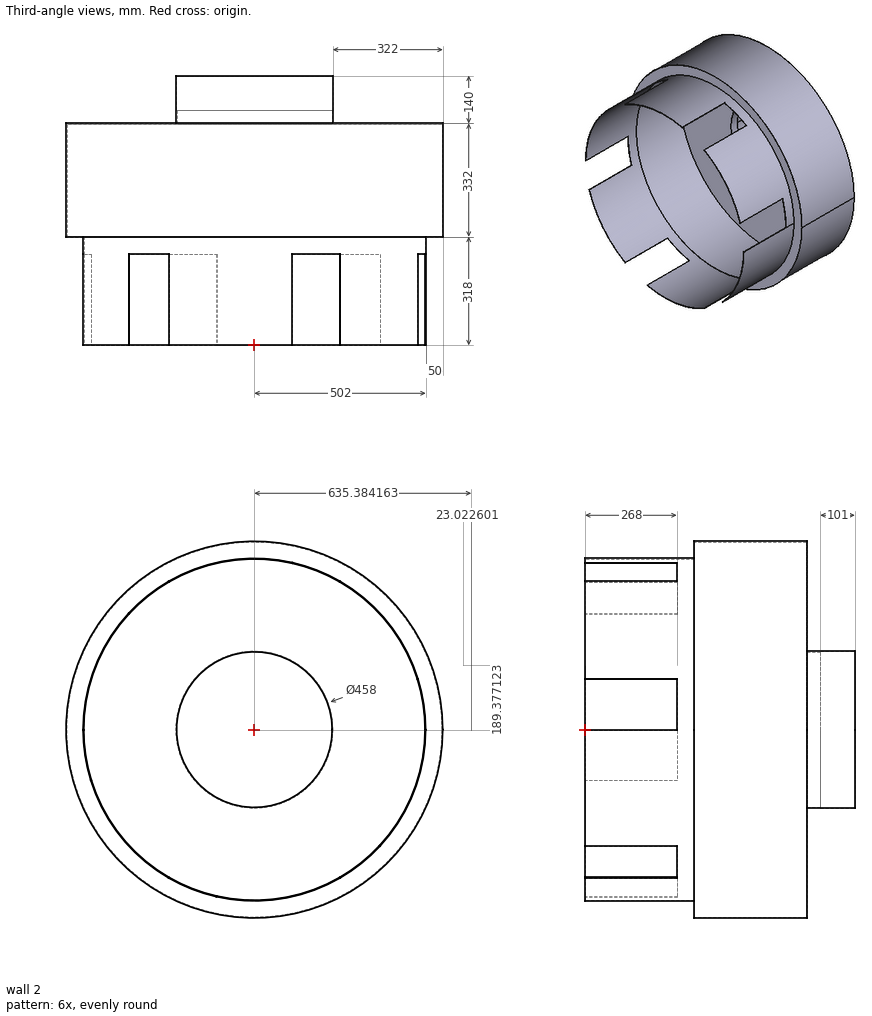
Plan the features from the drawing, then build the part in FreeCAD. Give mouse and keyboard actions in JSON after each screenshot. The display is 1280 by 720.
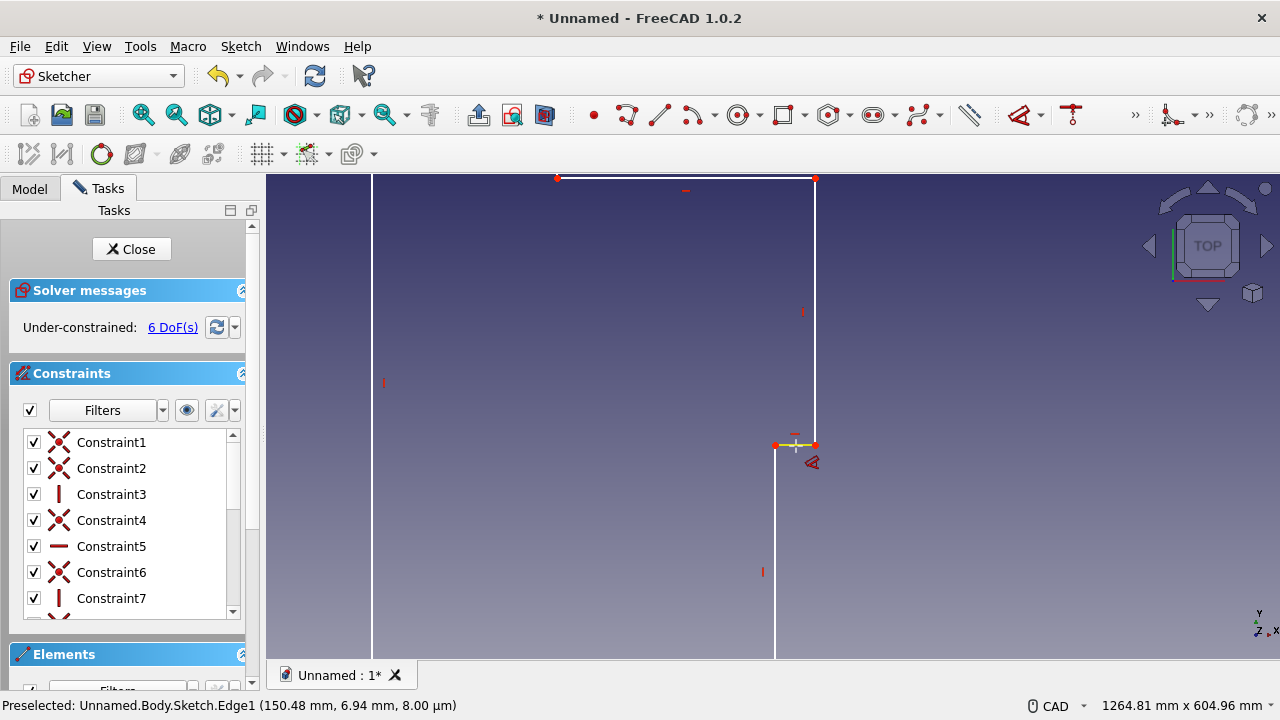
{"action": "left_click", "coordinate": [795, 445]}
{"action": "left_click", "coordinate": [795, 479]}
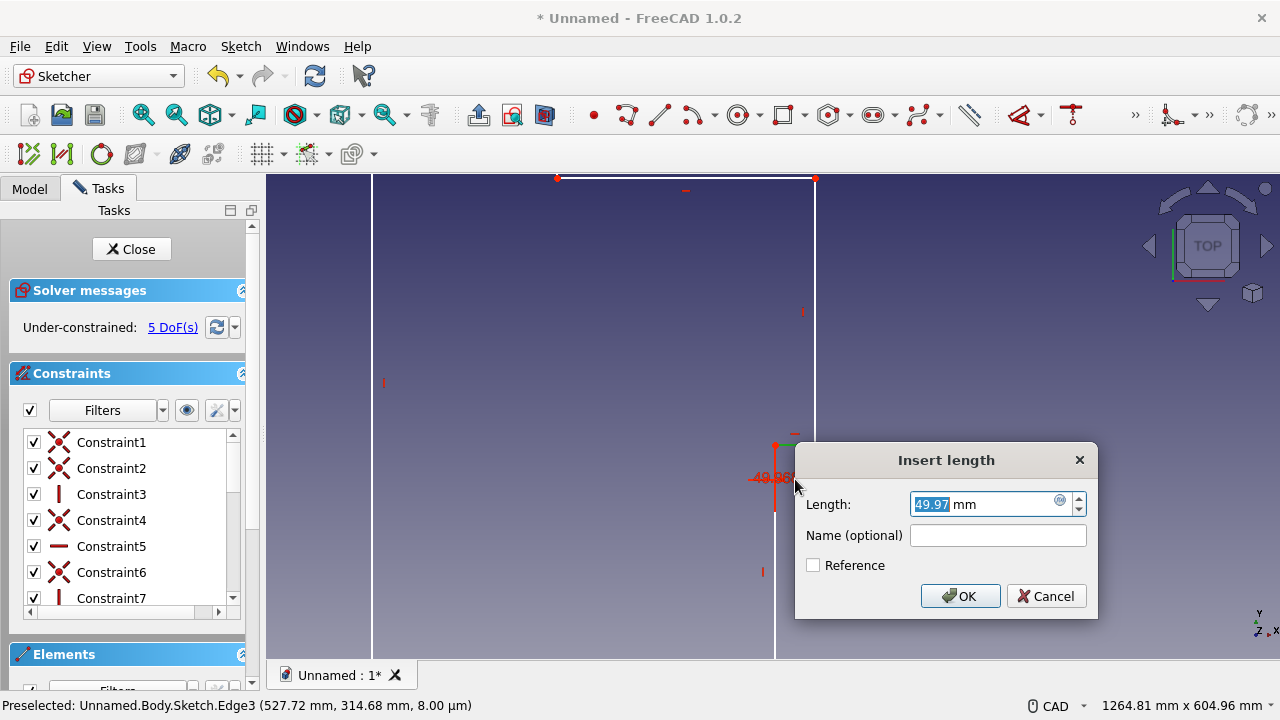
{"action": "type", "text": "50"}
{"action": "key", "text": "Return"}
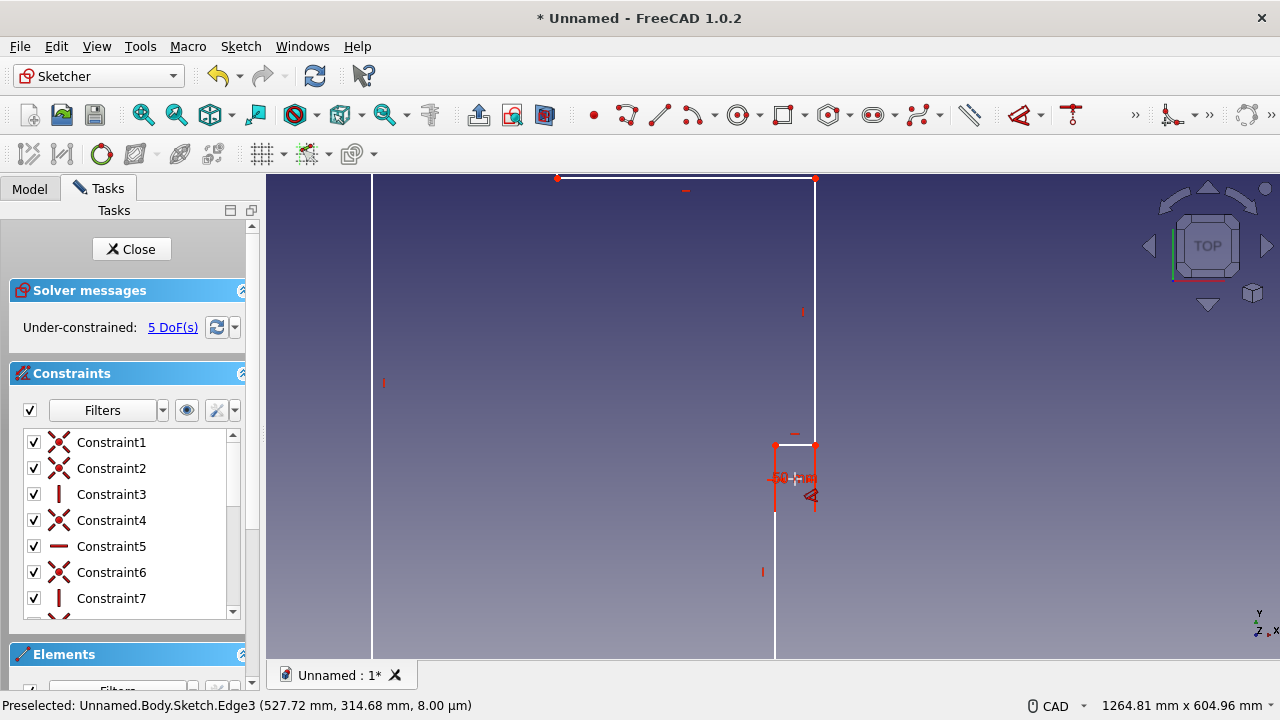
{"action": "scroll", "coordinate": [795, 446], "scroll_direction": "down", "scroll_amount": 4}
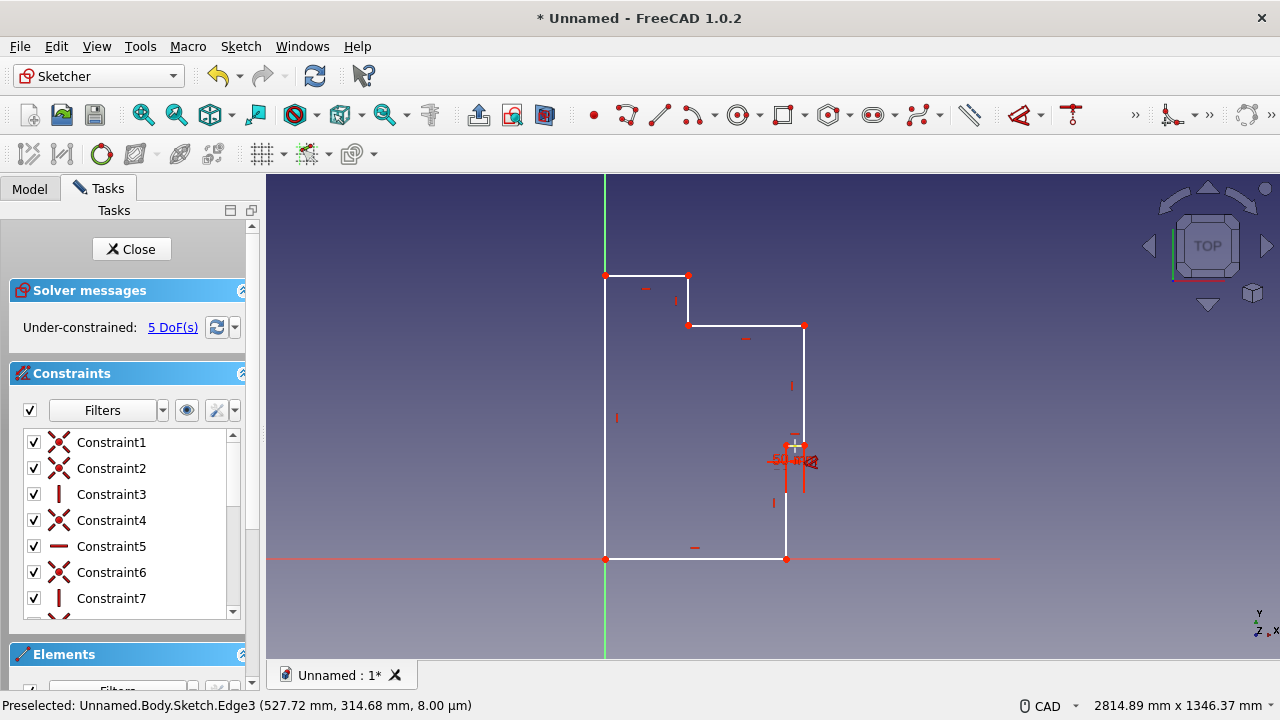
{"action": "left_click", "coordinate": [660, 559]}
{"action": "left_click", "coordinate": [696, 593]}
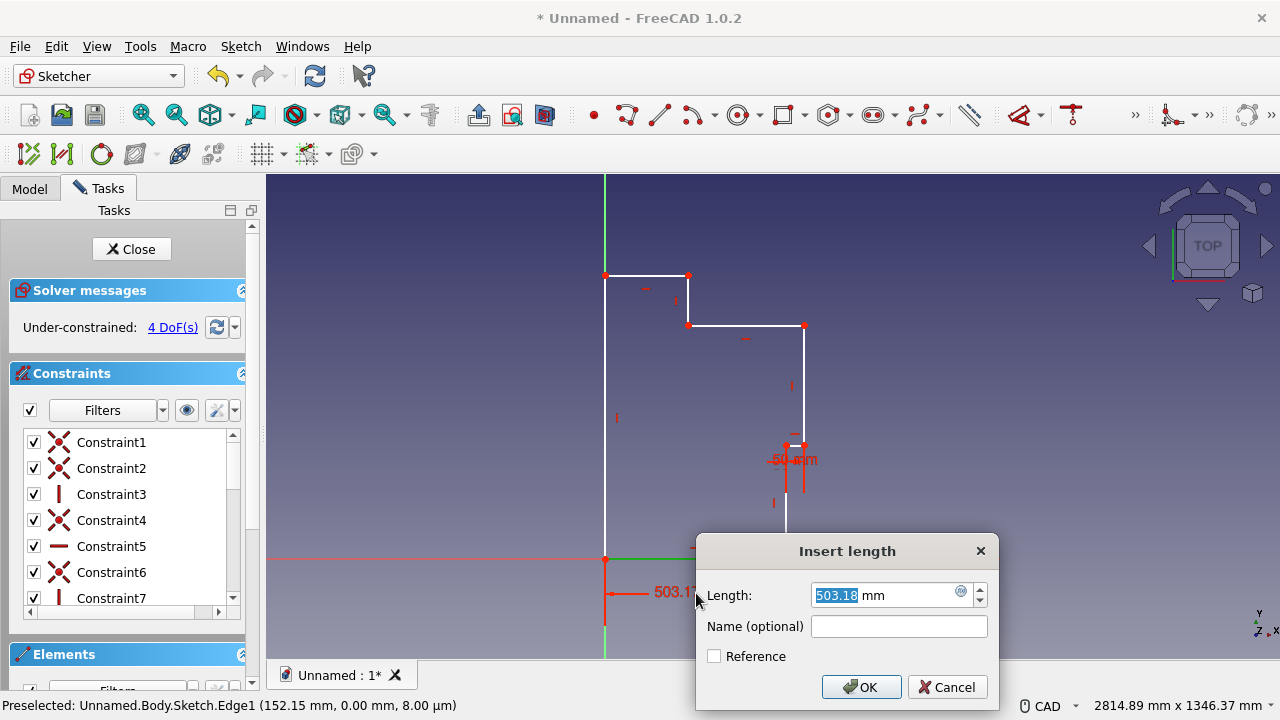
{"action": "type", "text": "502"}
{"action": "key", "text": "Return"}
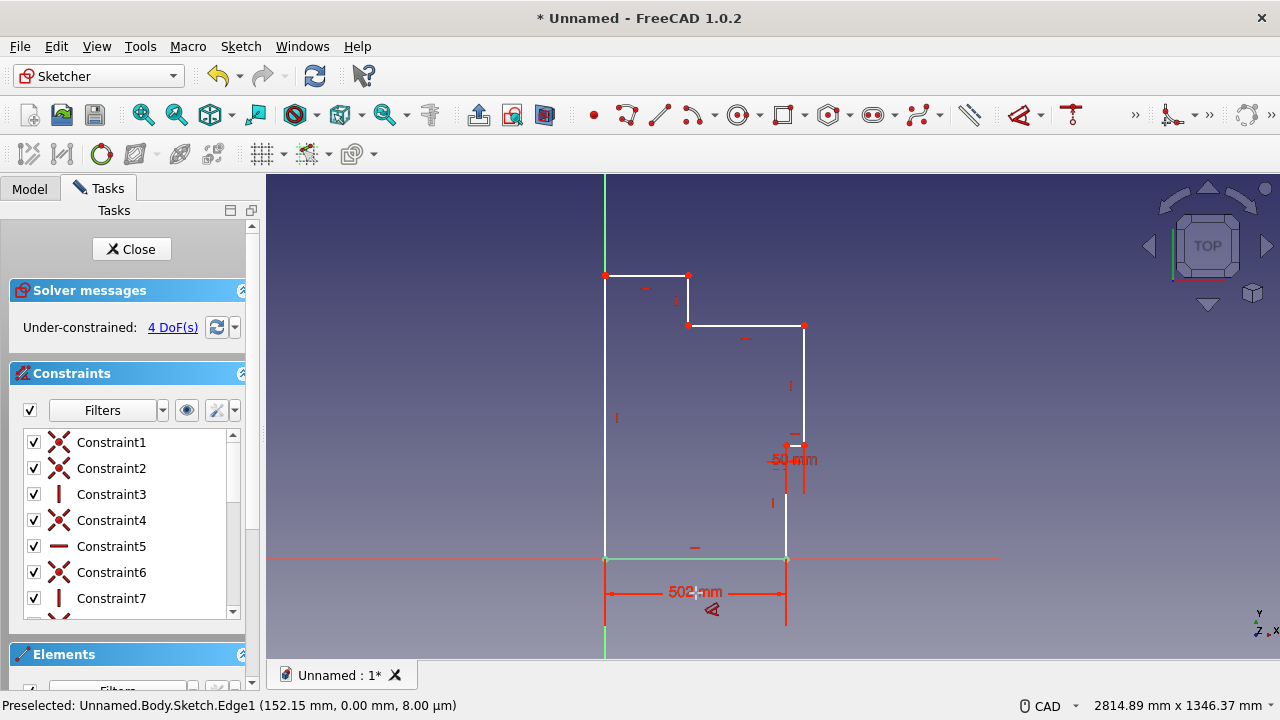
{"action": "left_click", "coordinate": [786, 525]}
{"action": "left_click", "coordinate": [820, 503]}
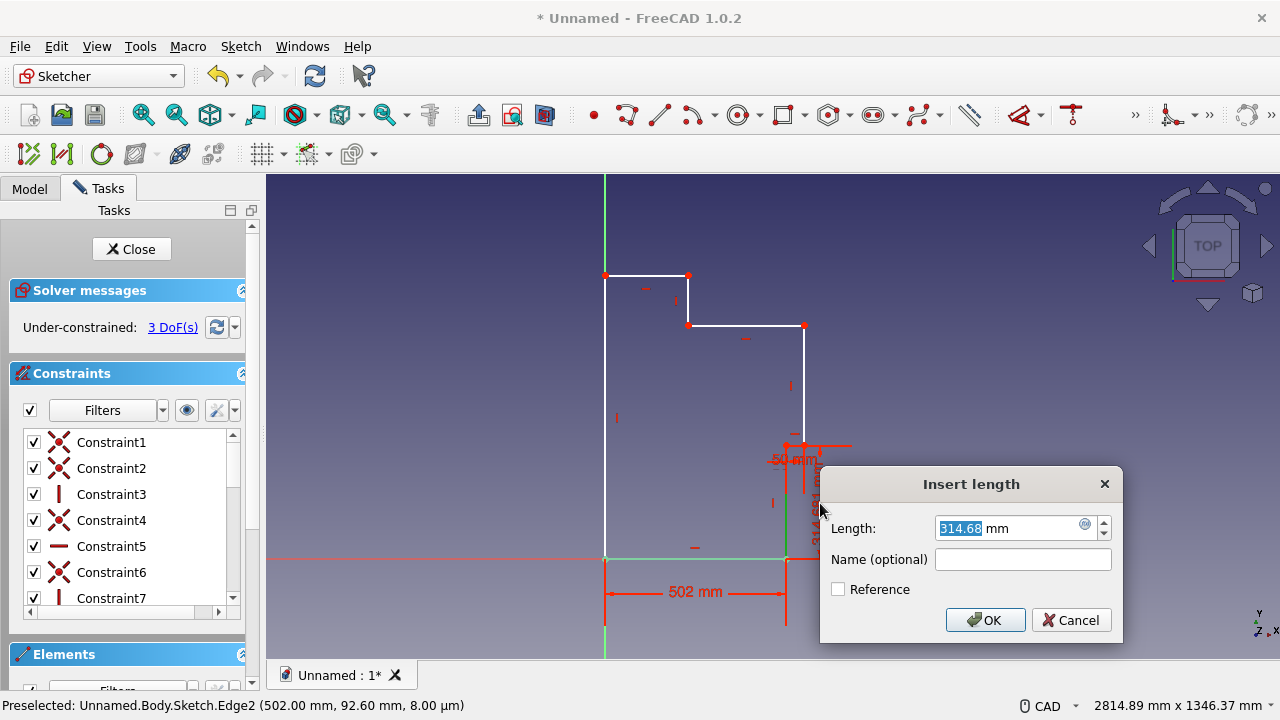
{"action": "type", "text": "318"}
{"action": "key", "text": "Return"}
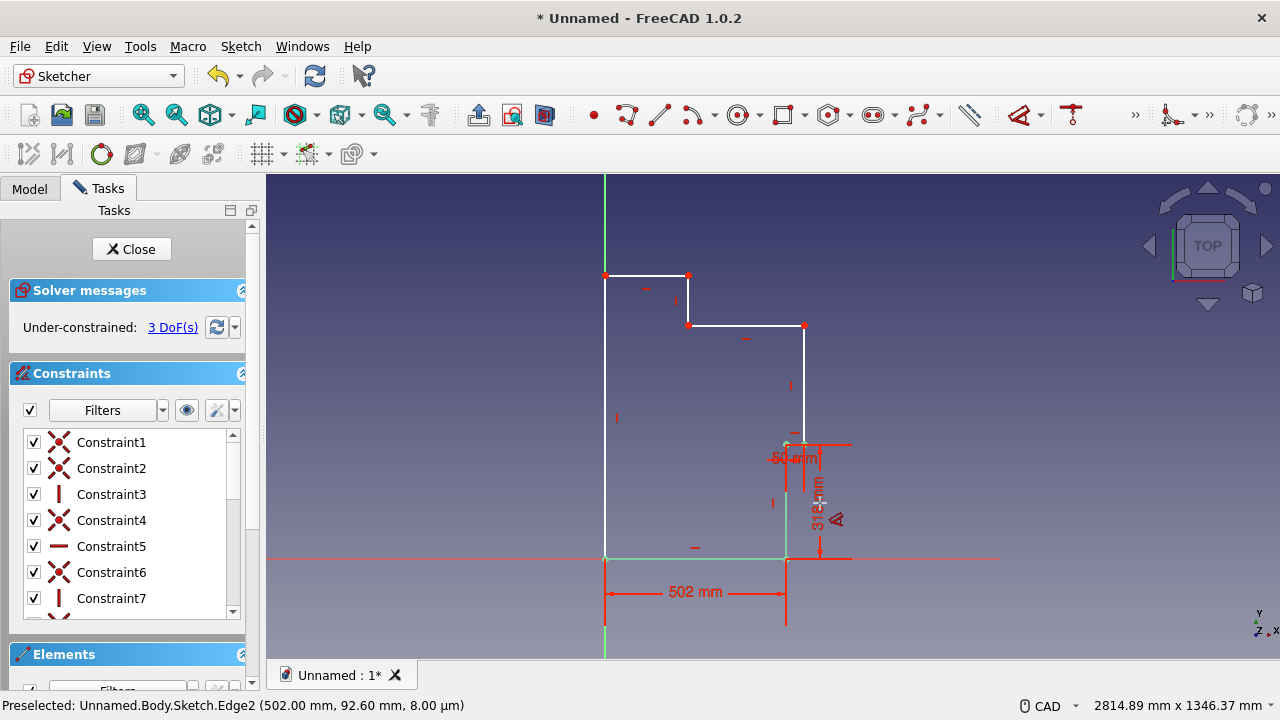
{"action": "left_click", "coordinate": [804, 409]}
{"action": "left_click", "coordinate": [838, 385]}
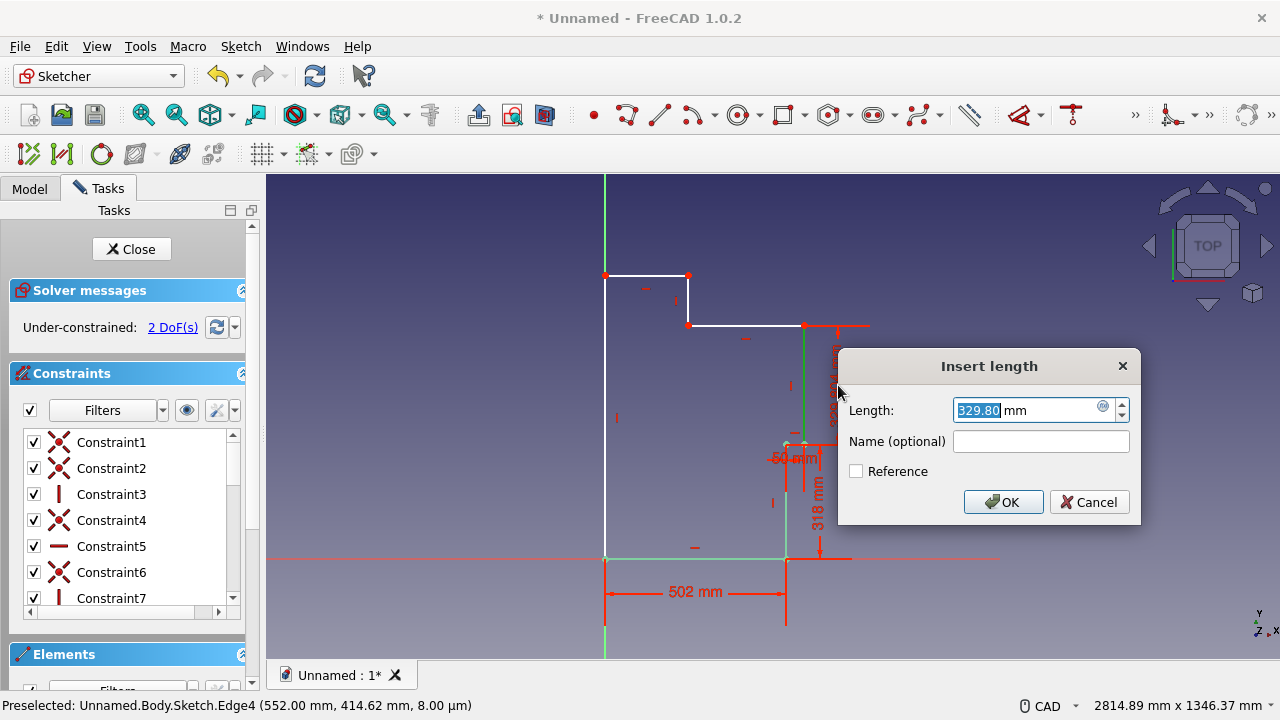
{"action": "type", "text": "332"}
{"action": "key", "text": "Return"}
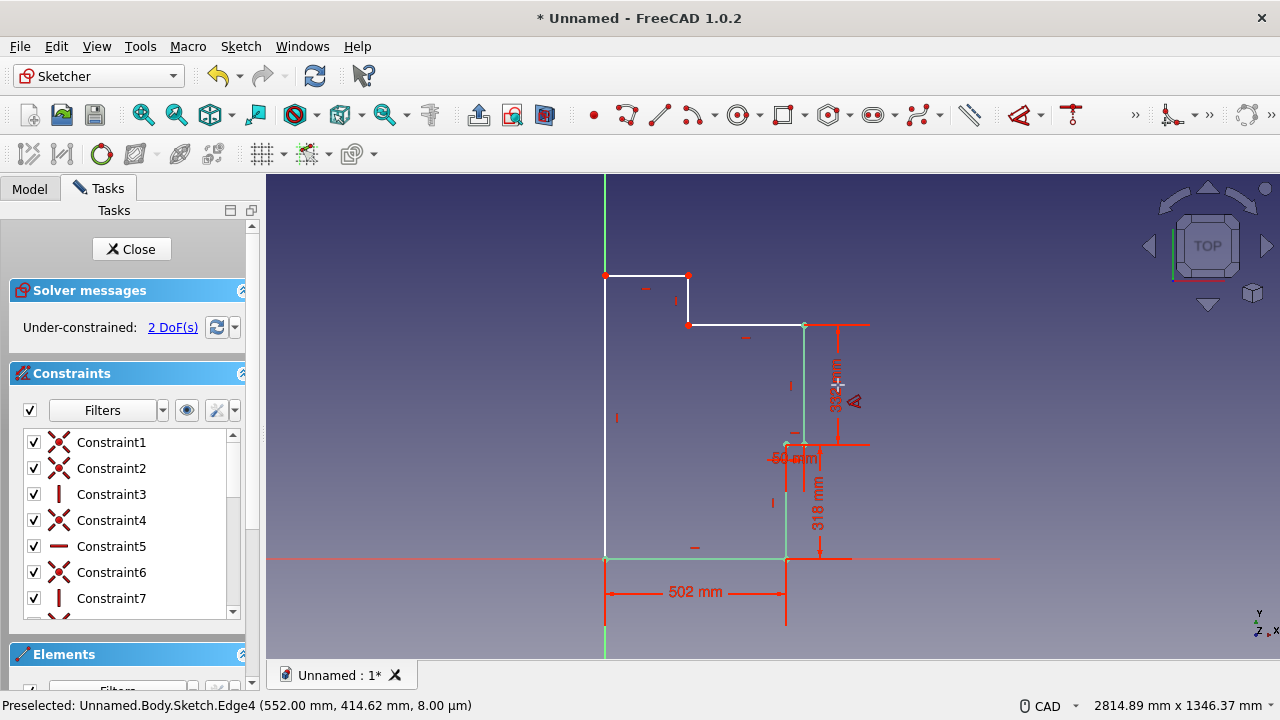
{"action": "left_click", "coordinate": [769, 325]}
{"action": "left_click", "coordinate": [746, 291]}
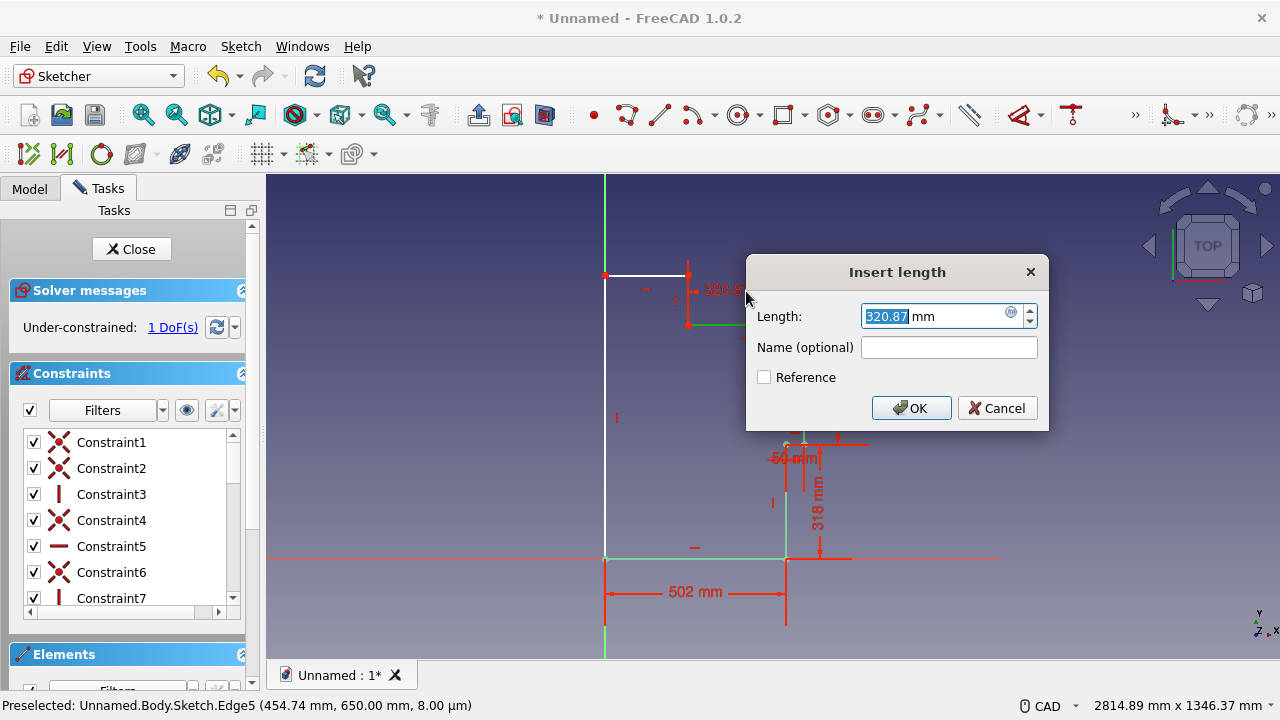
{"action": "type", "text": "322"}
{"action": "key", "text": "Return"}